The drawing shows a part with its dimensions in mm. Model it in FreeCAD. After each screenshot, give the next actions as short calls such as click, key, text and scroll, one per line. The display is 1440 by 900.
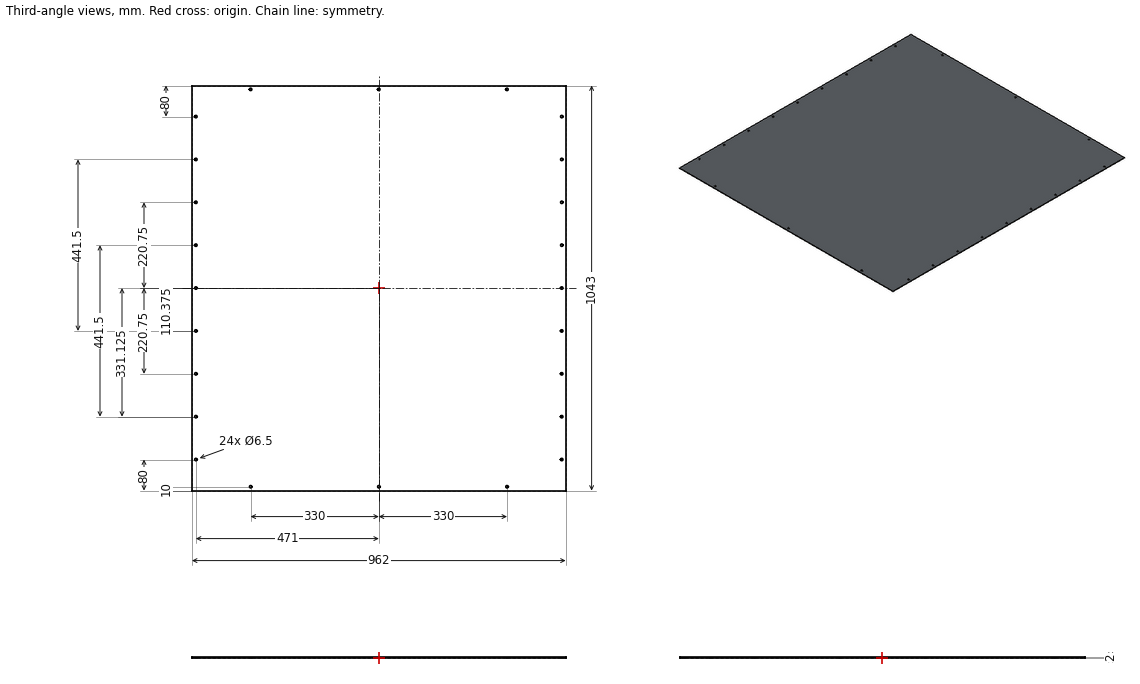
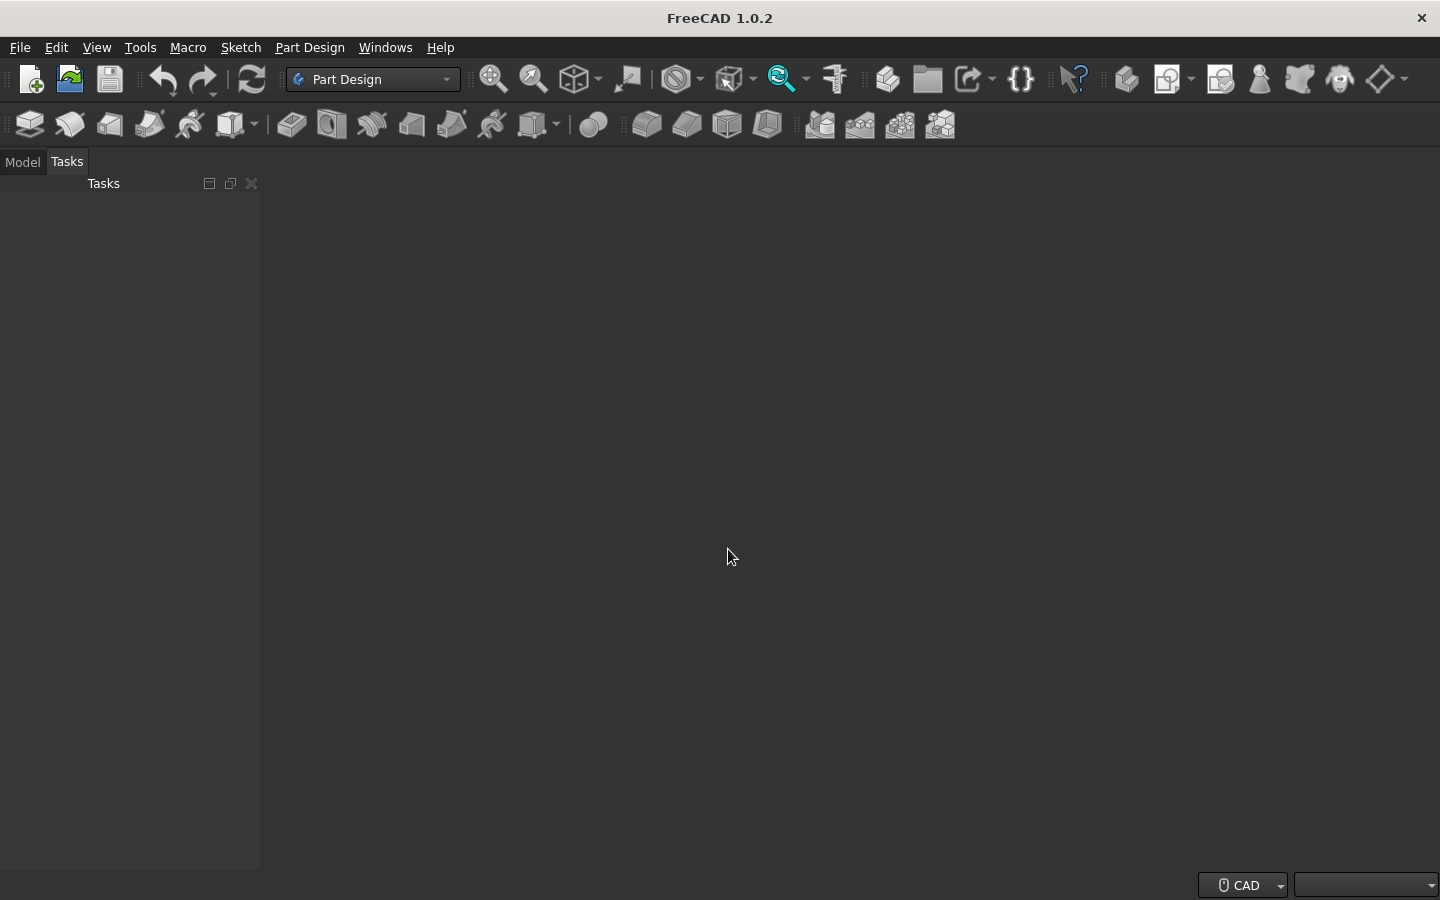
click(30, 80)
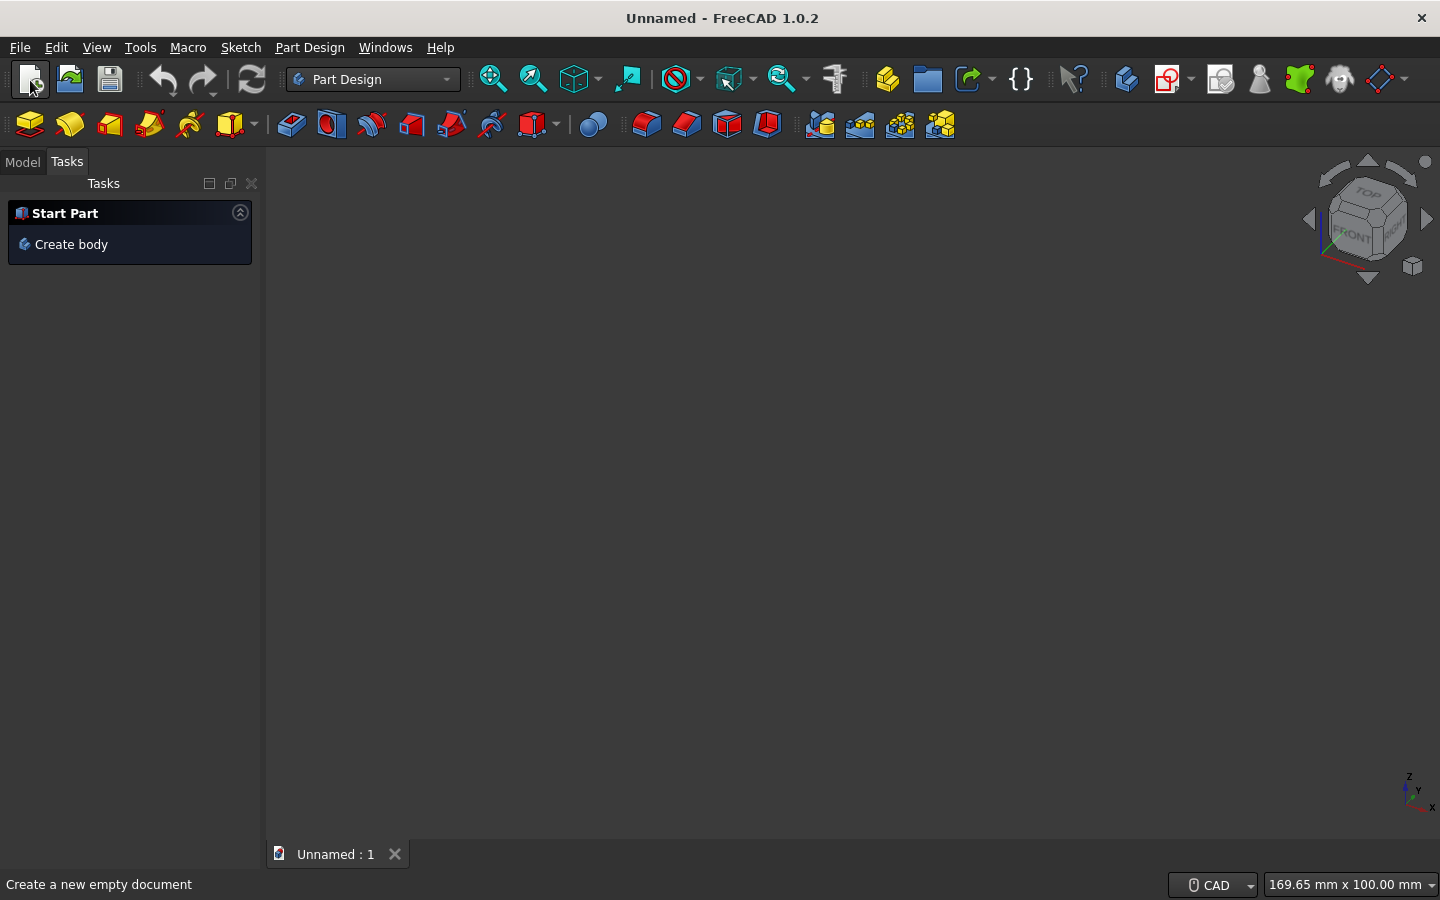
click(1168, 80)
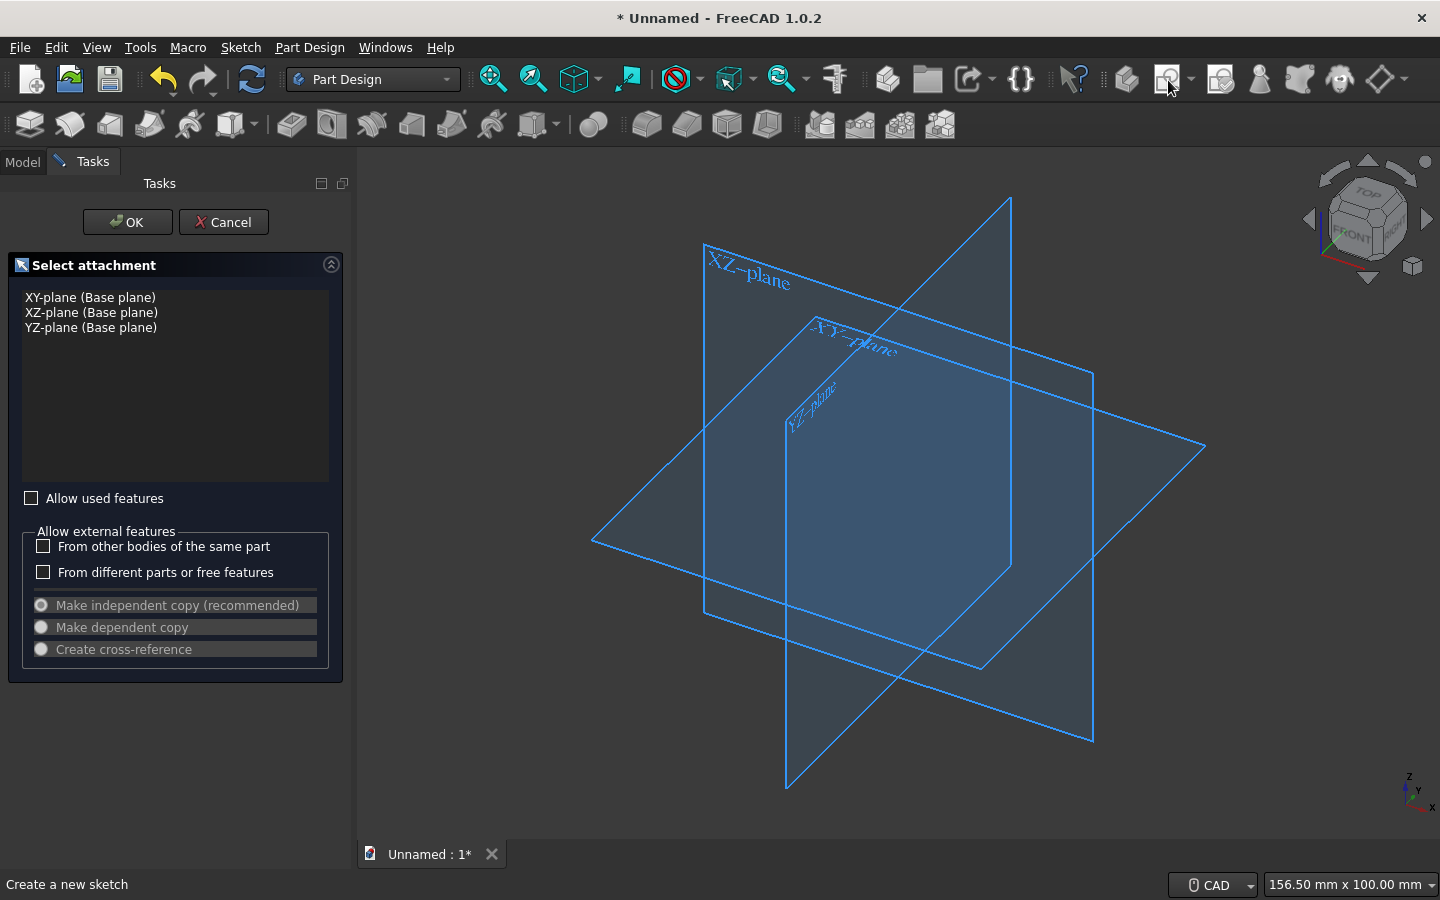
click(82, 298)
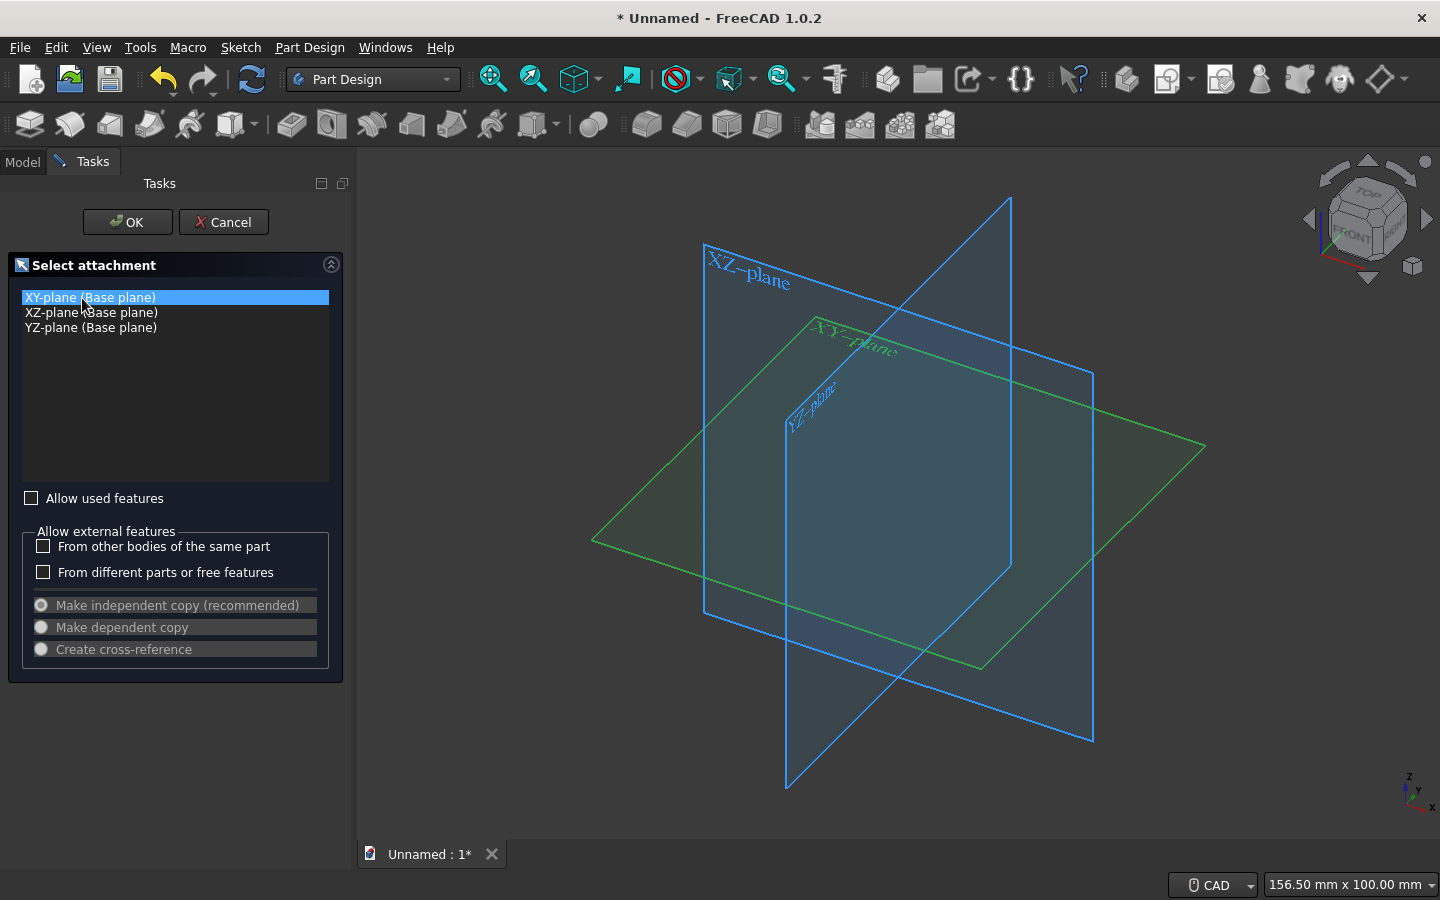
click(128, 222)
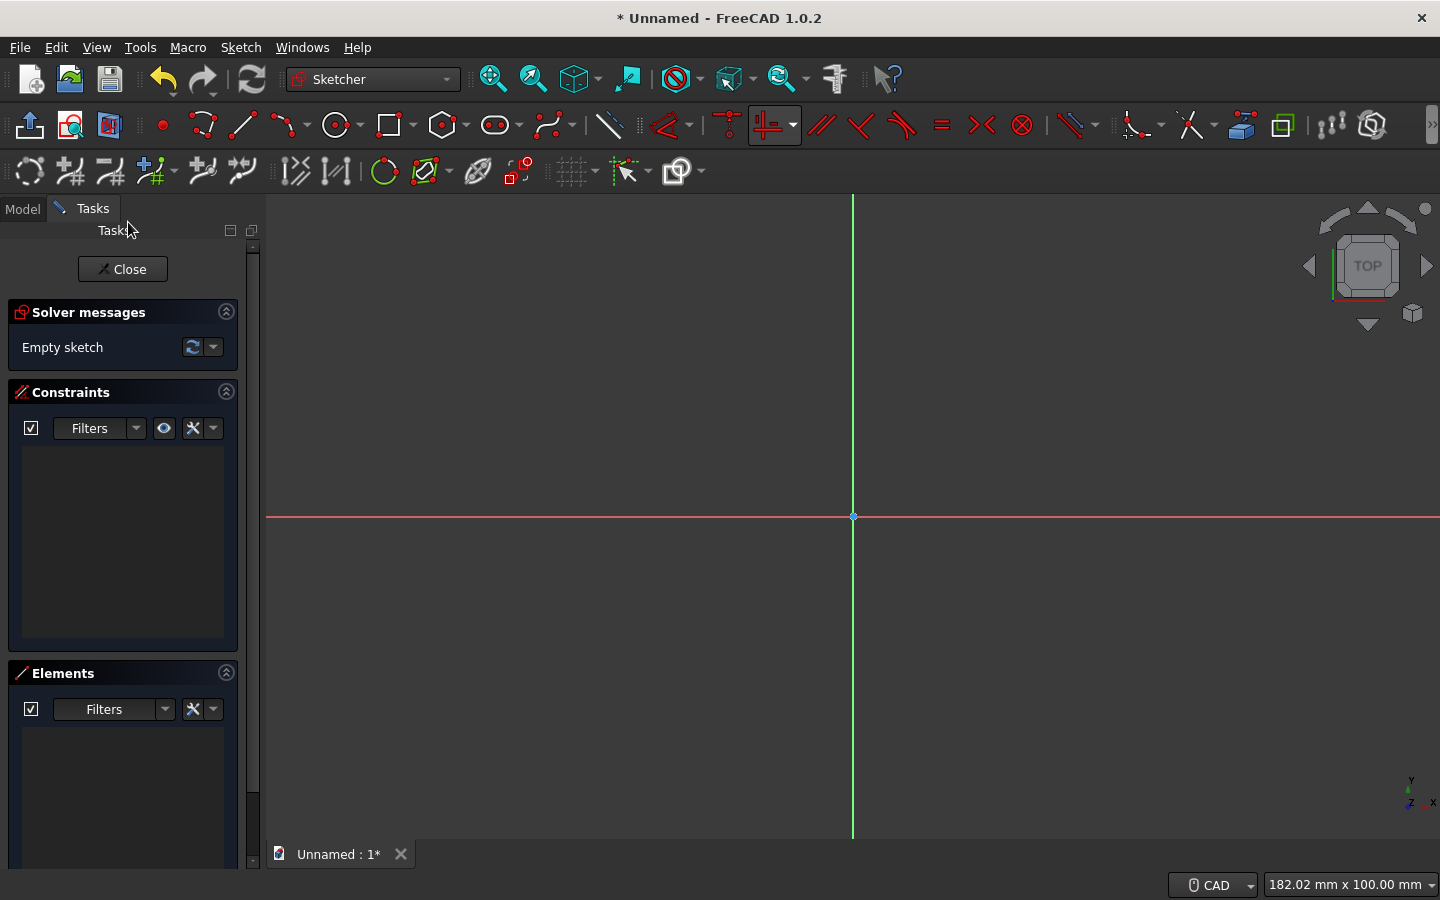
scroll(780, 516, down, 14)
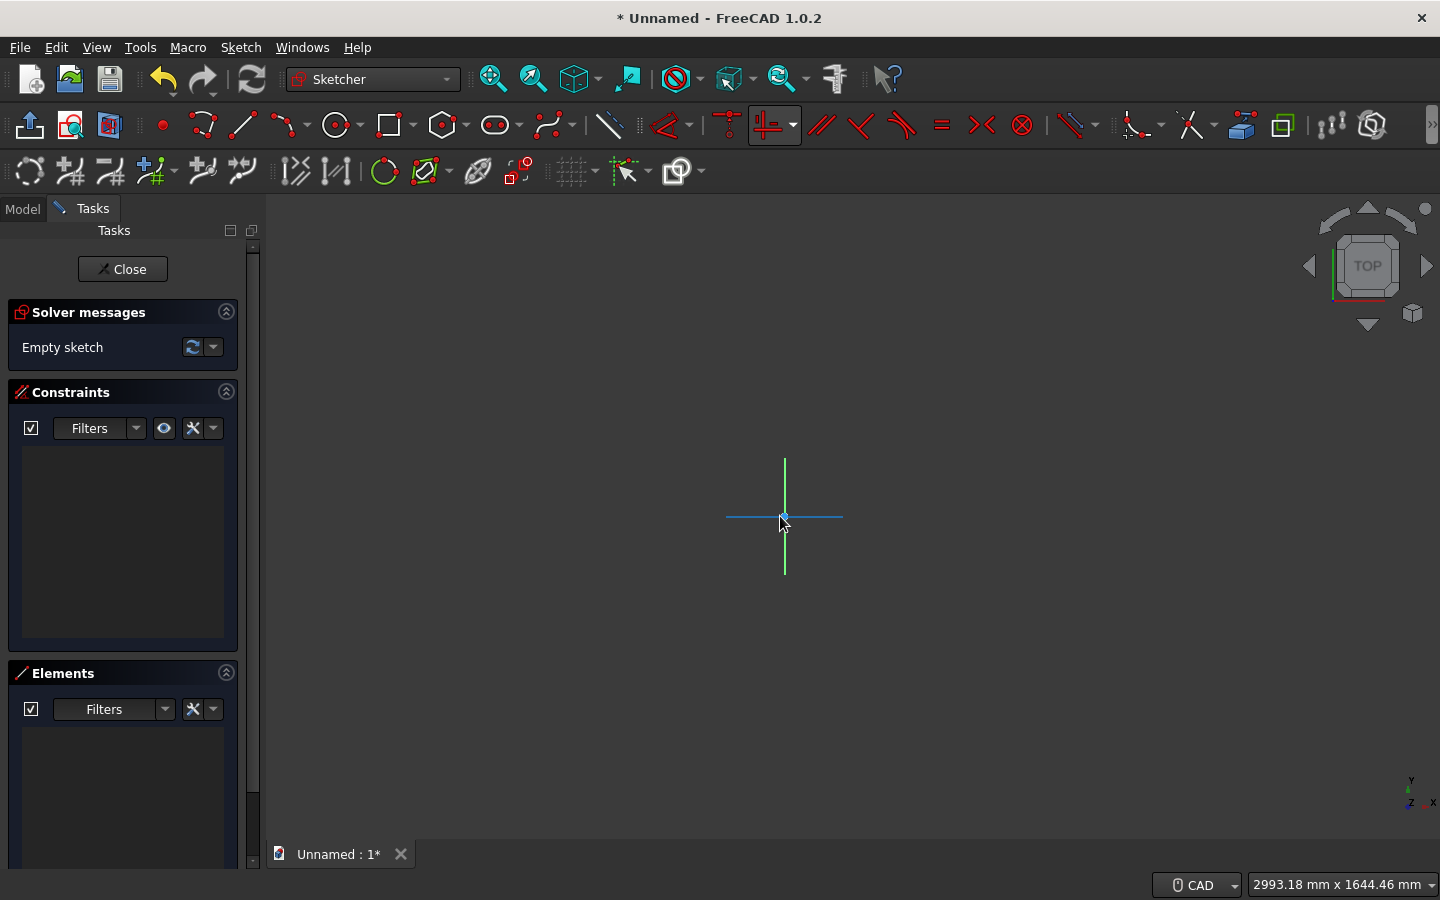
key(g)
key(v)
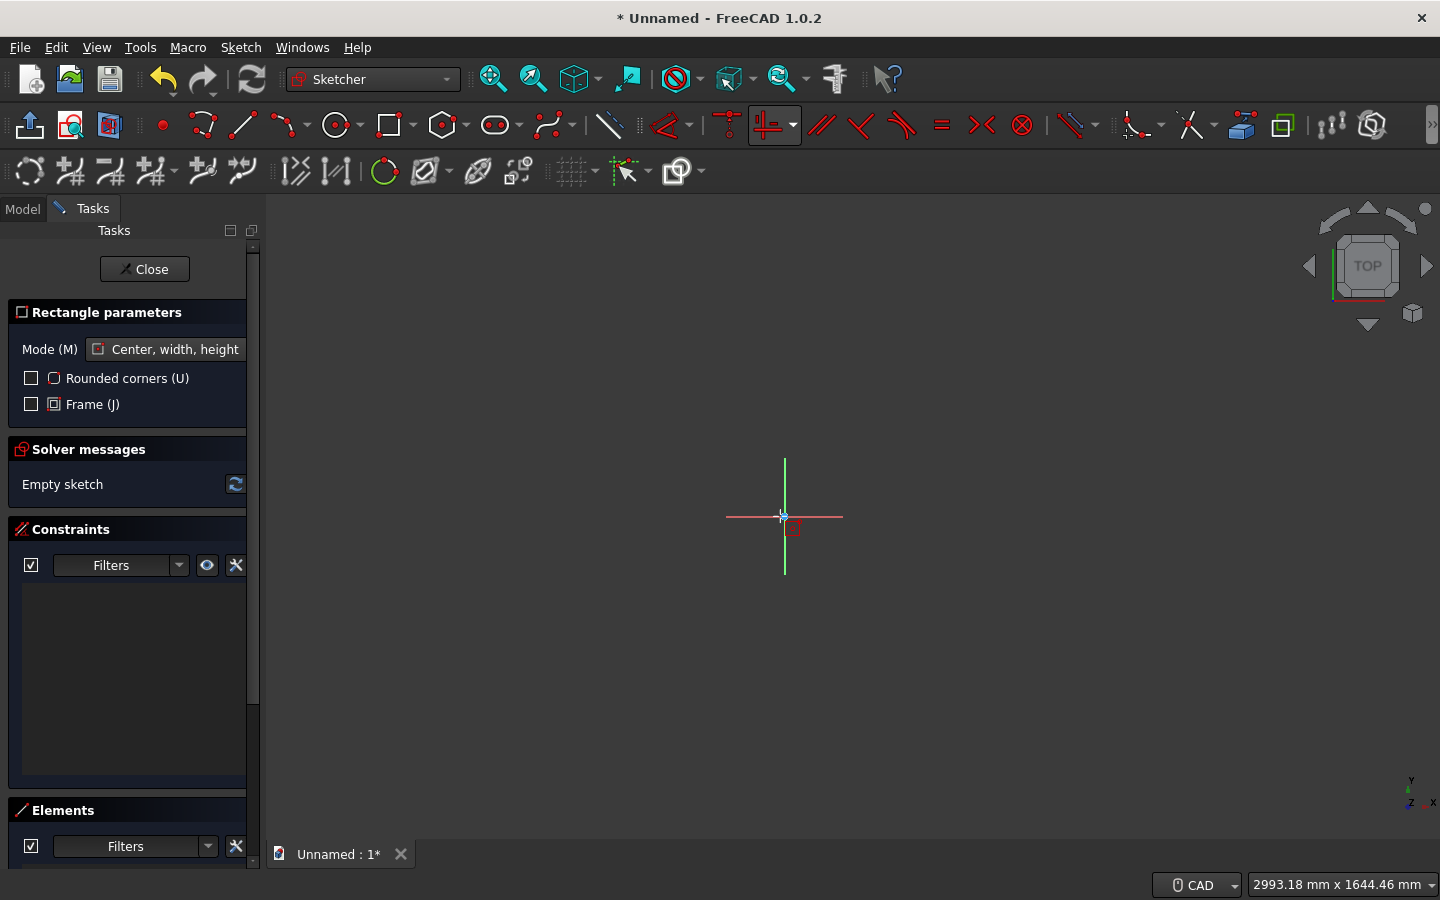
click(785, 516)
move(974, 312)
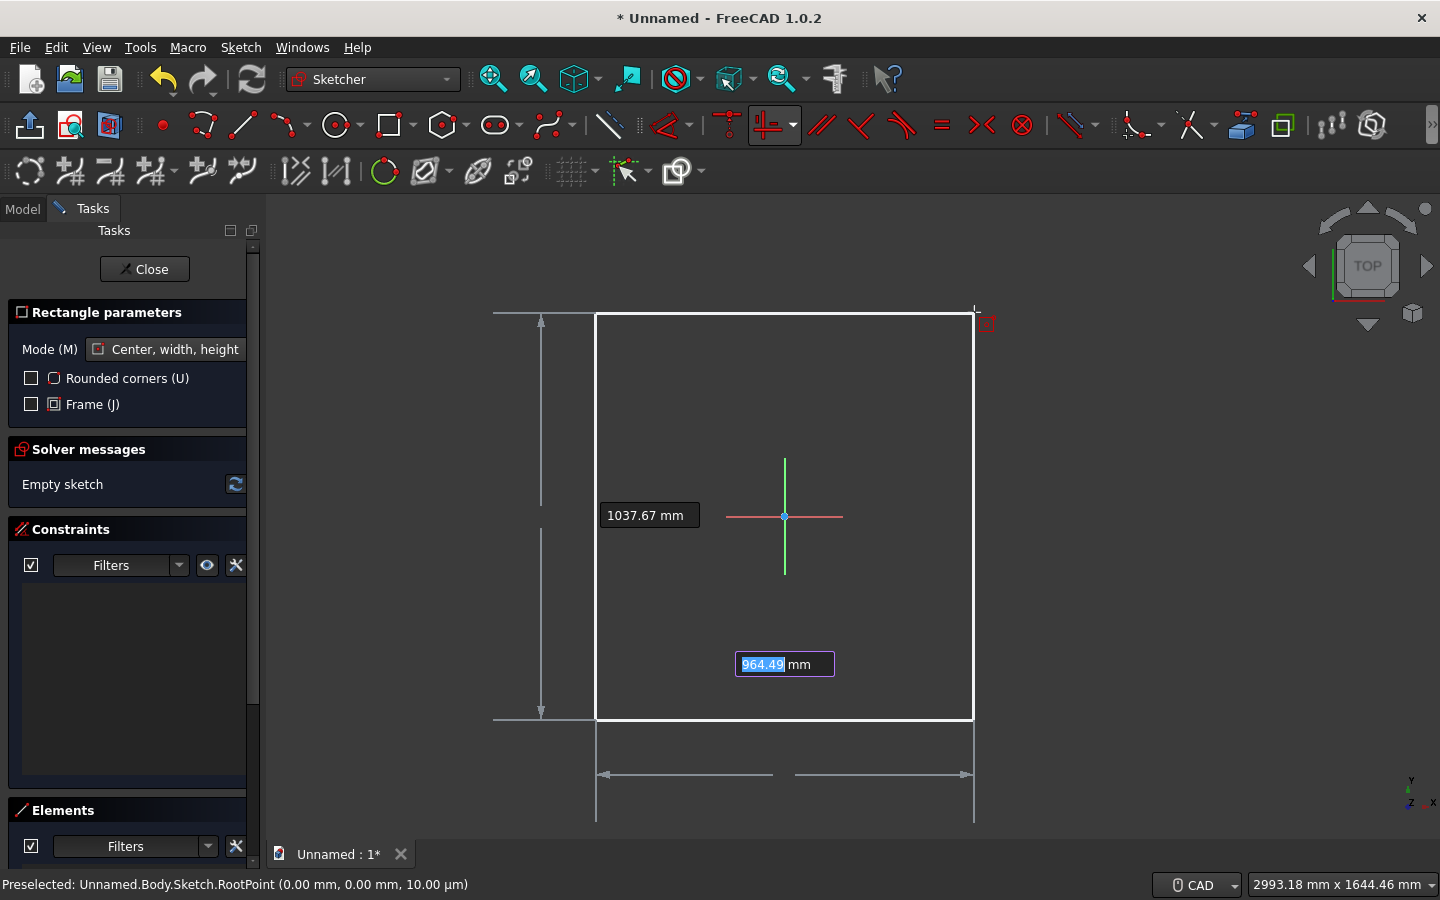
text(962)
key(Tab)
text(1043)
key(Return)